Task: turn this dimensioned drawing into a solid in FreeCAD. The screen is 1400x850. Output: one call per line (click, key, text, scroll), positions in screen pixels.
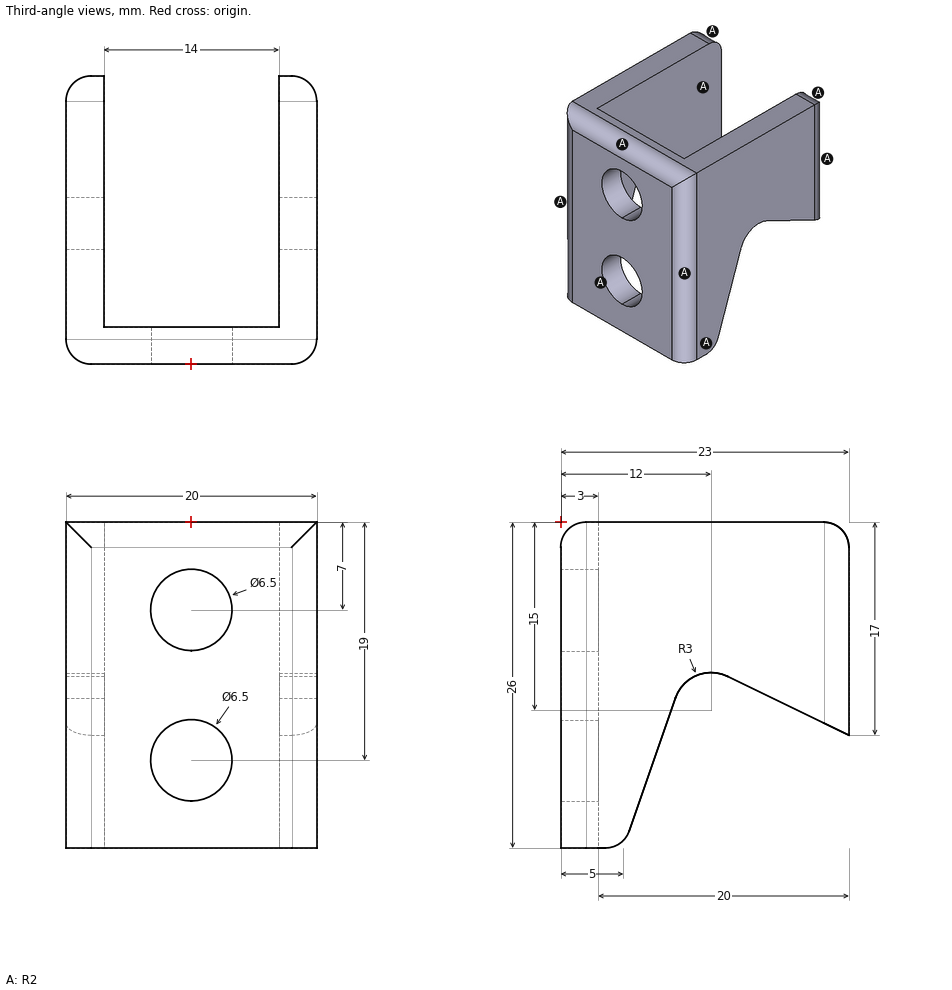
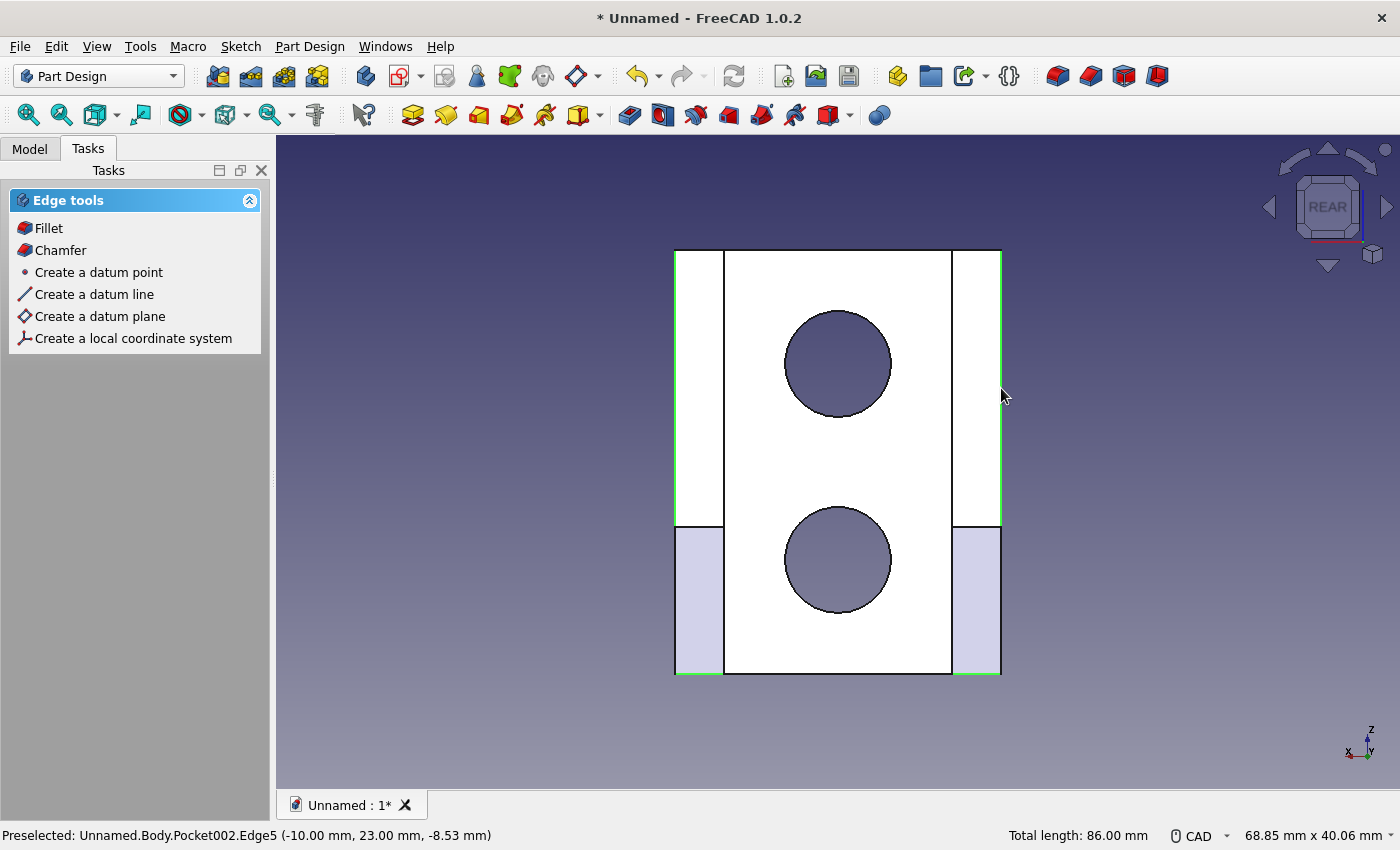
click(699, 249, ctrl)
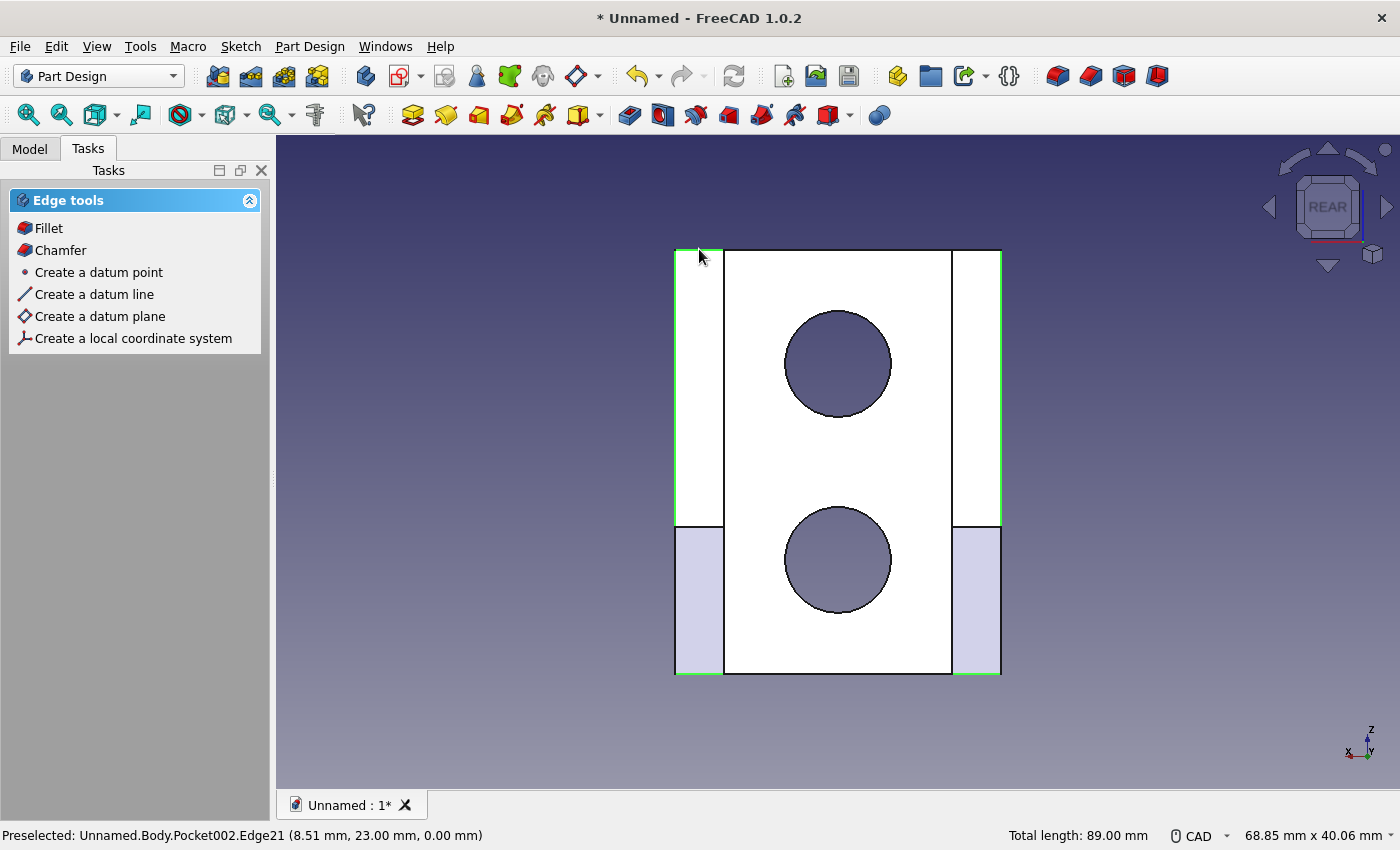
click(977, 249, ctrl)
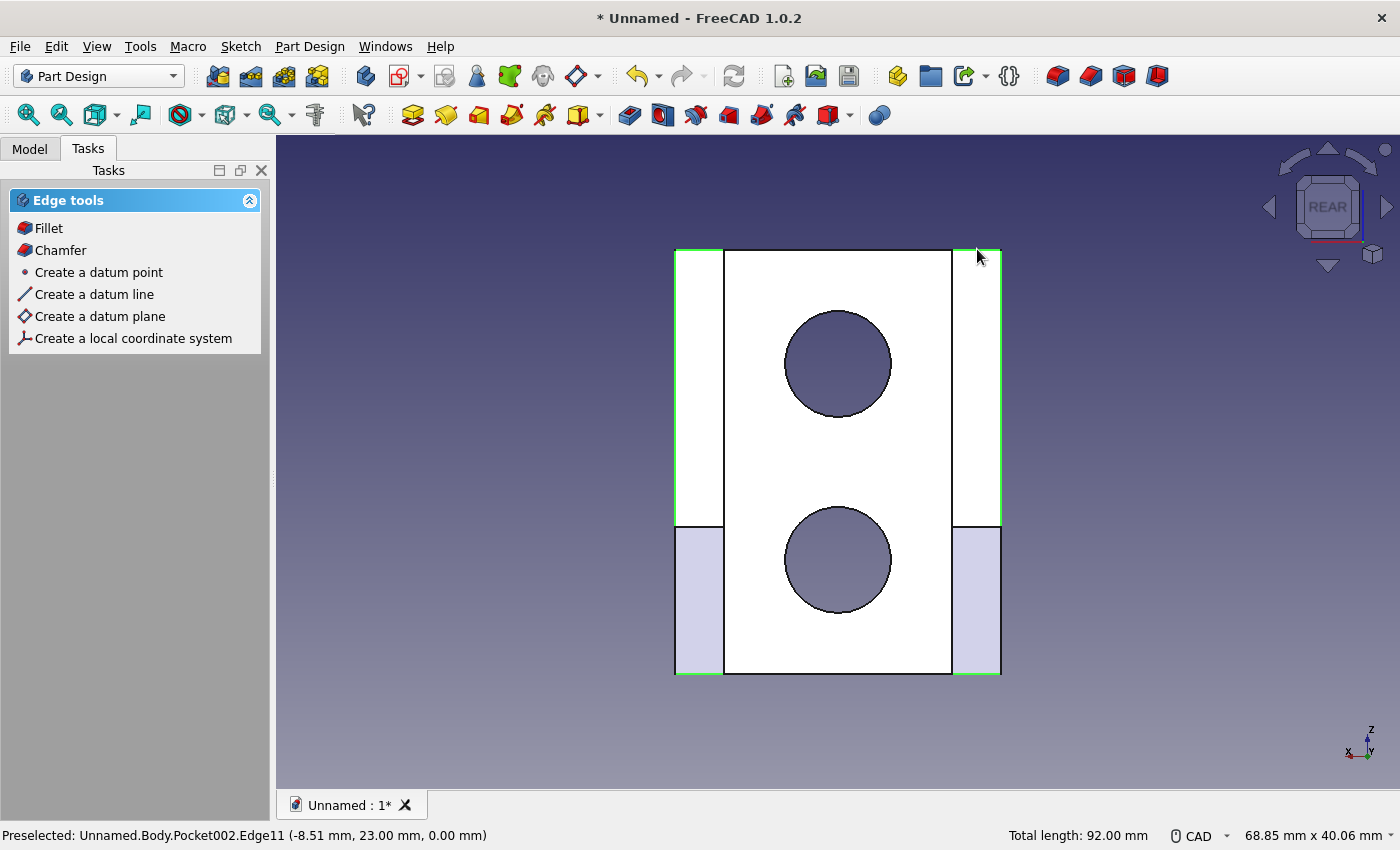
key(6)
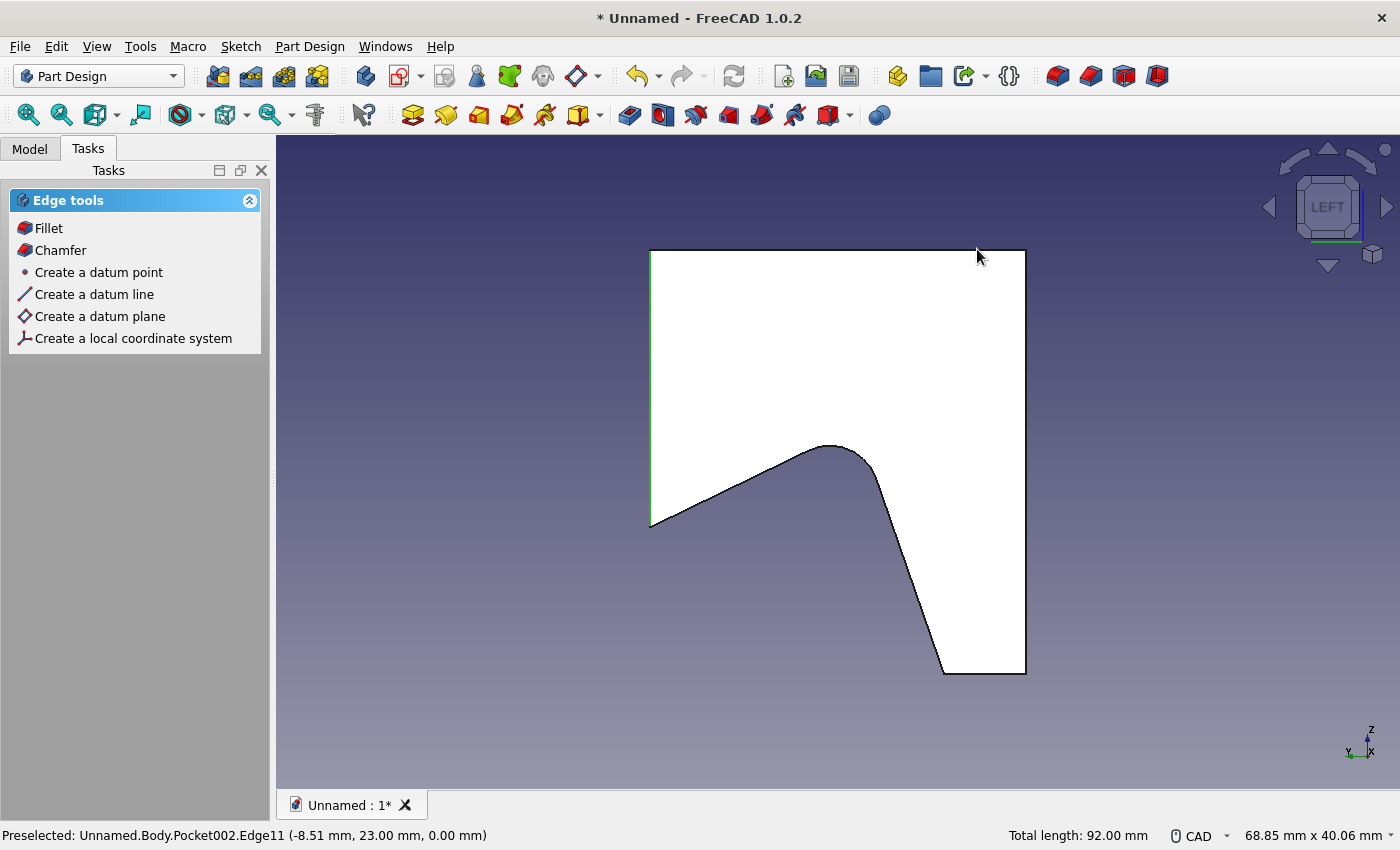
click(1026, 461, ctrl)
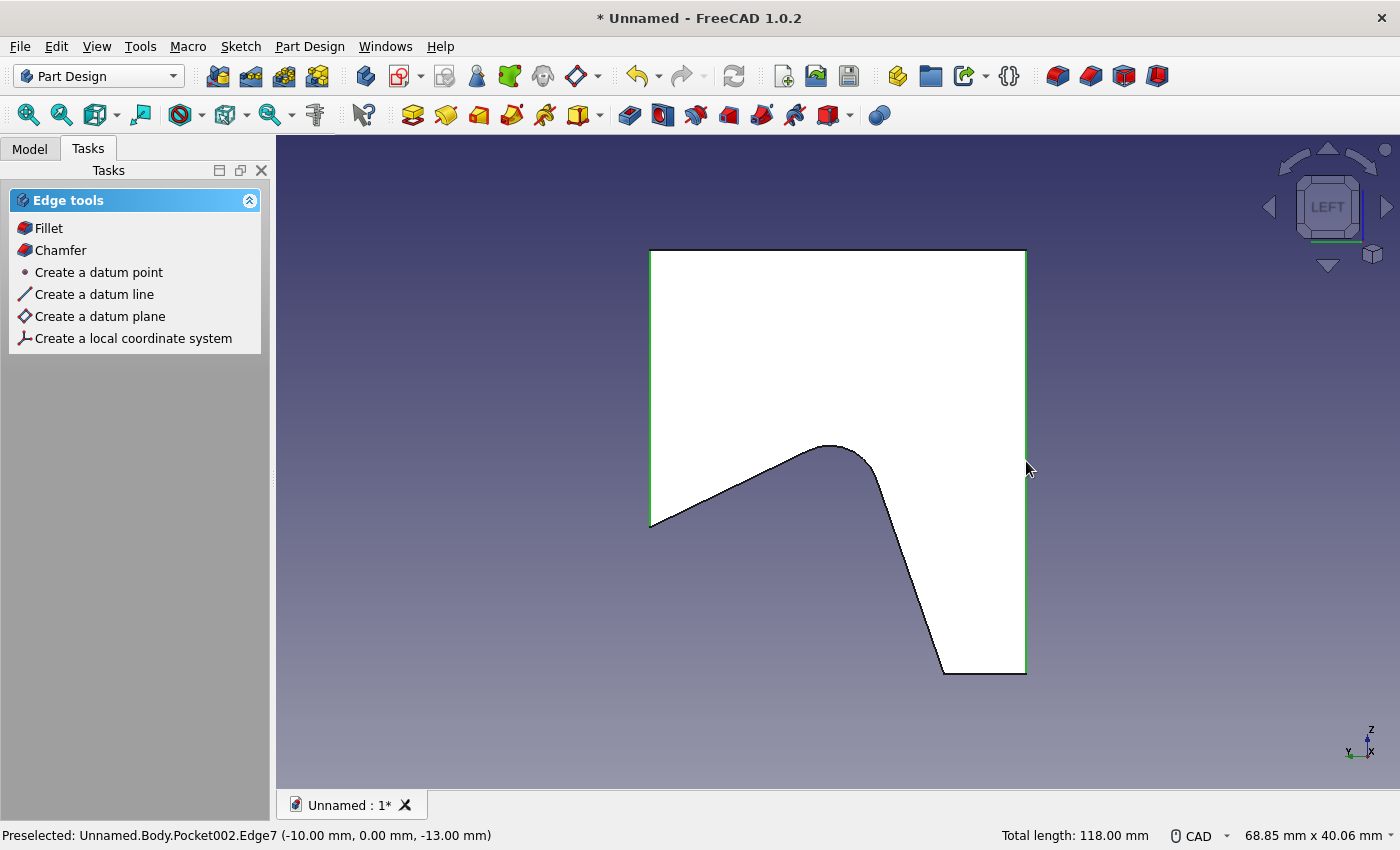
click(1058, 76)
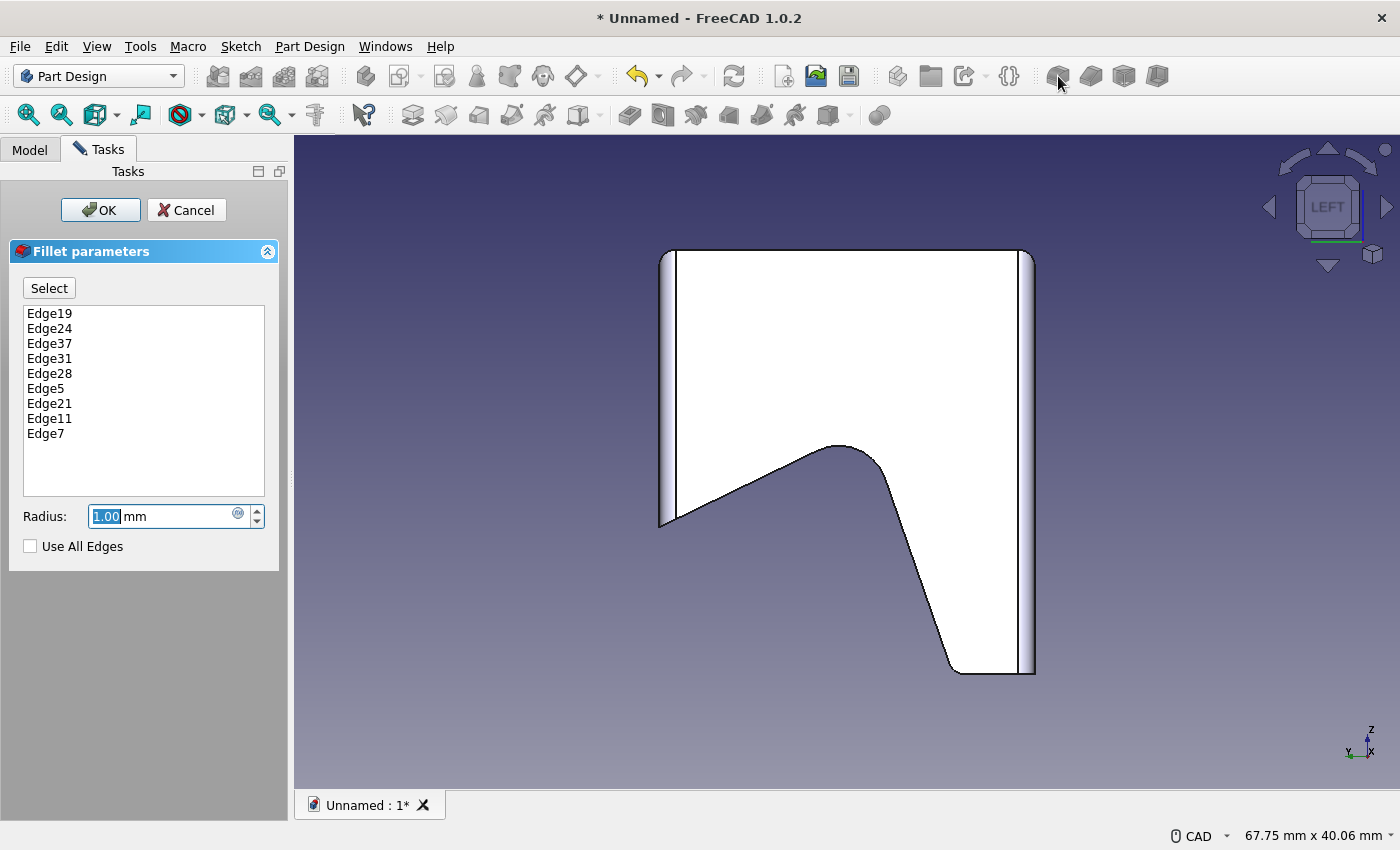
text(2)
key(Tab)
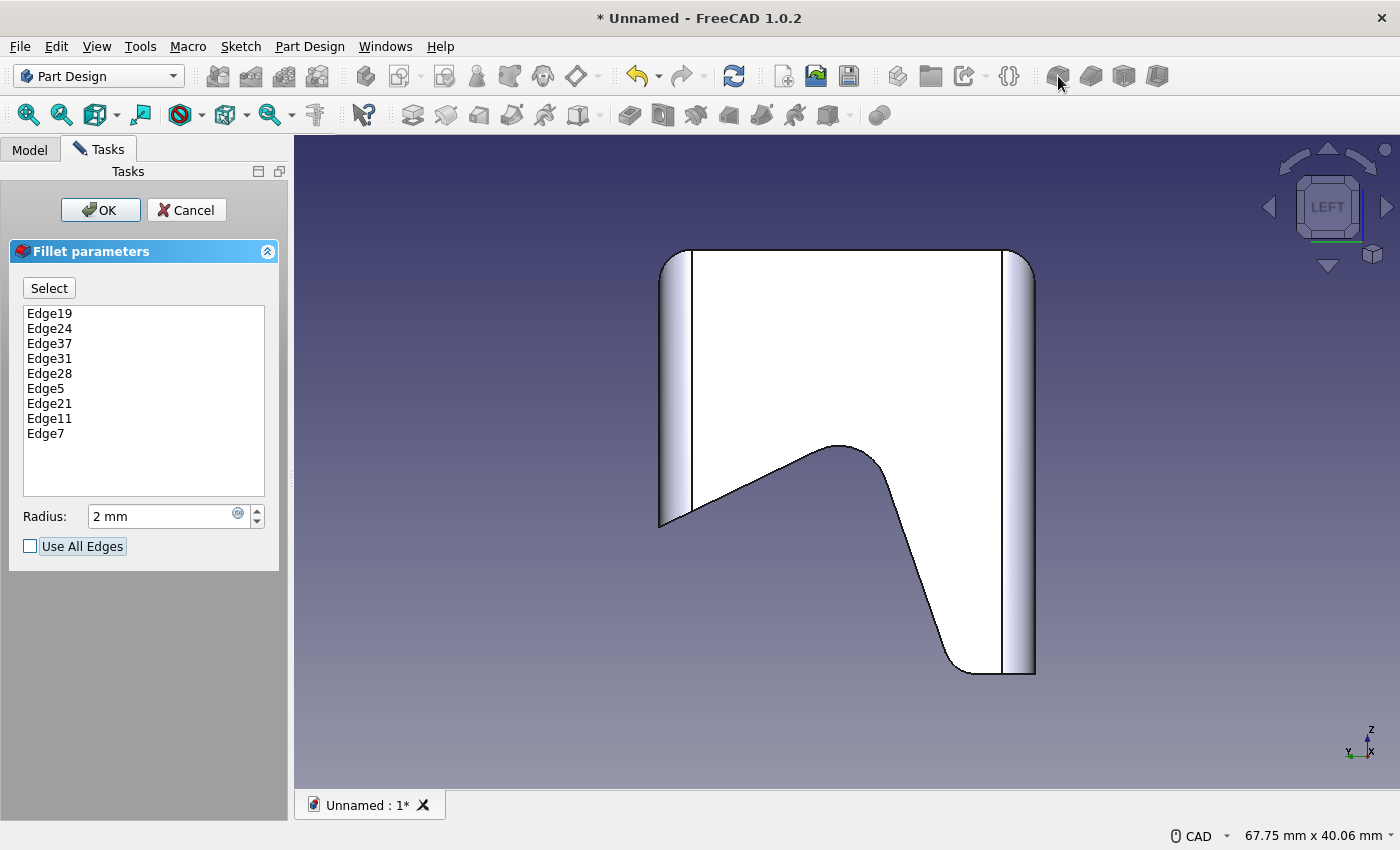
click(101, 210)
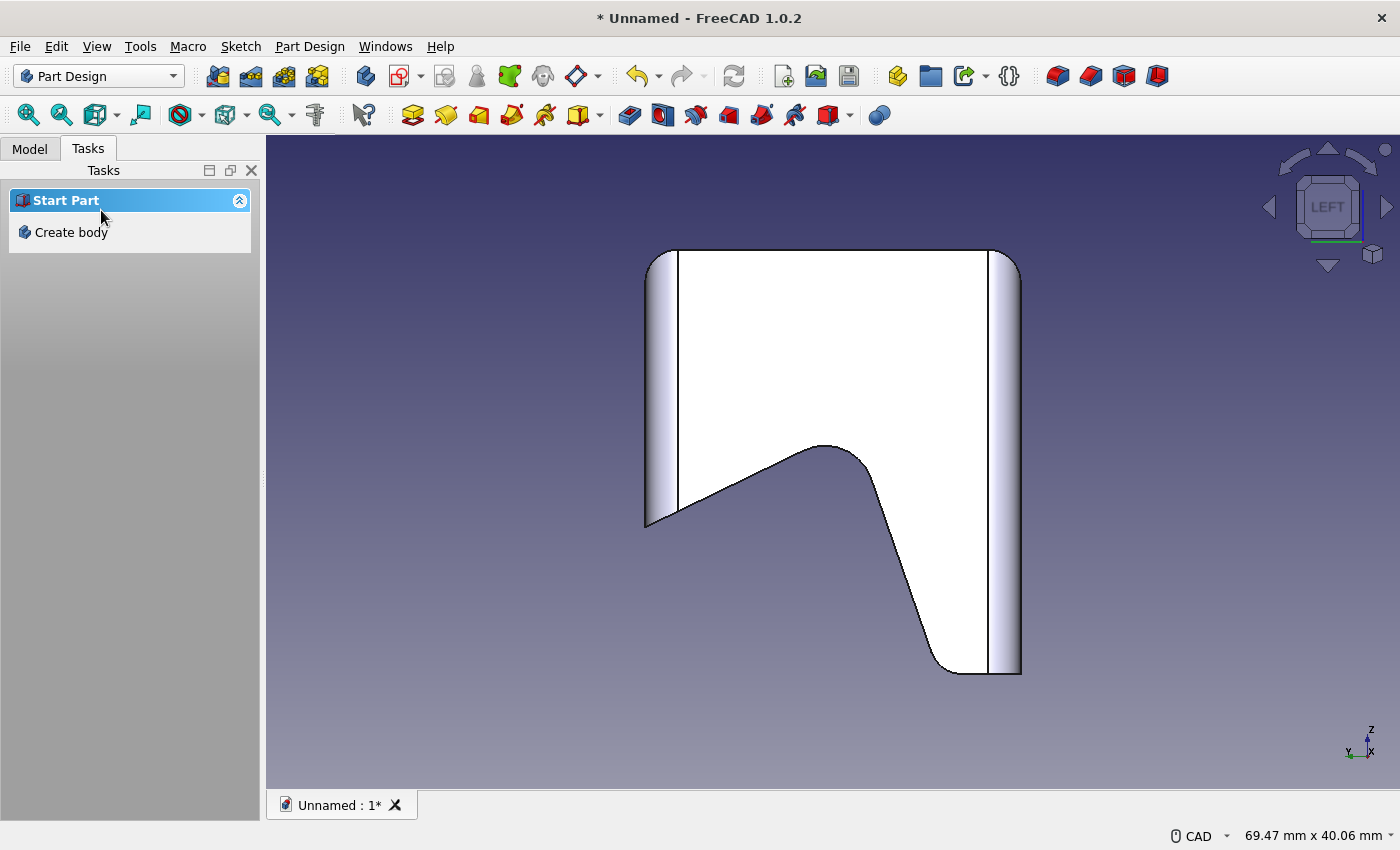
key(0)